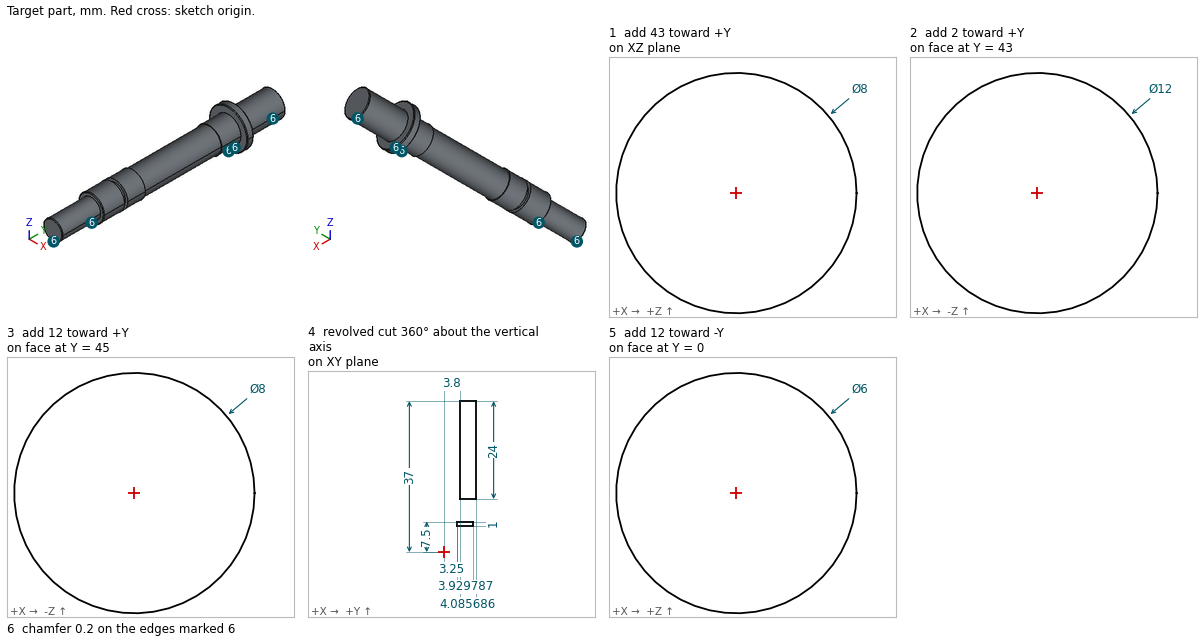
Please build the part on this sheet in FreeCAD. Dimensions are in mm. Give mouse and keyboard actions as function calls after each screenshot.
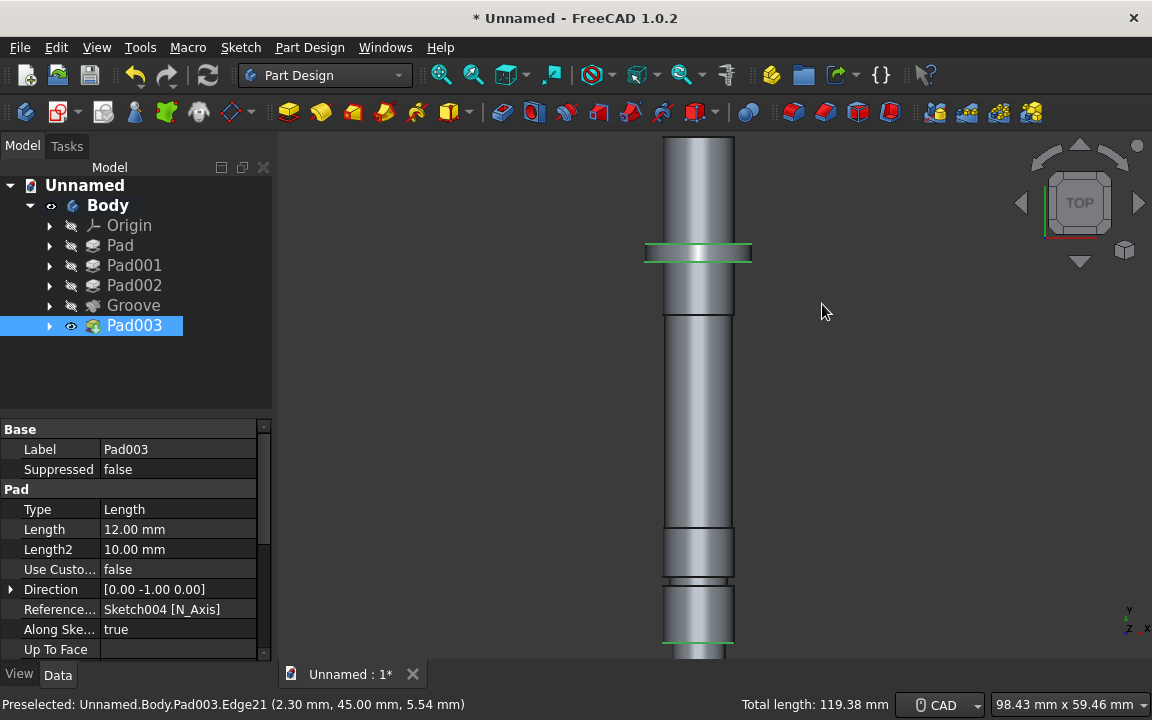
click(442, 76)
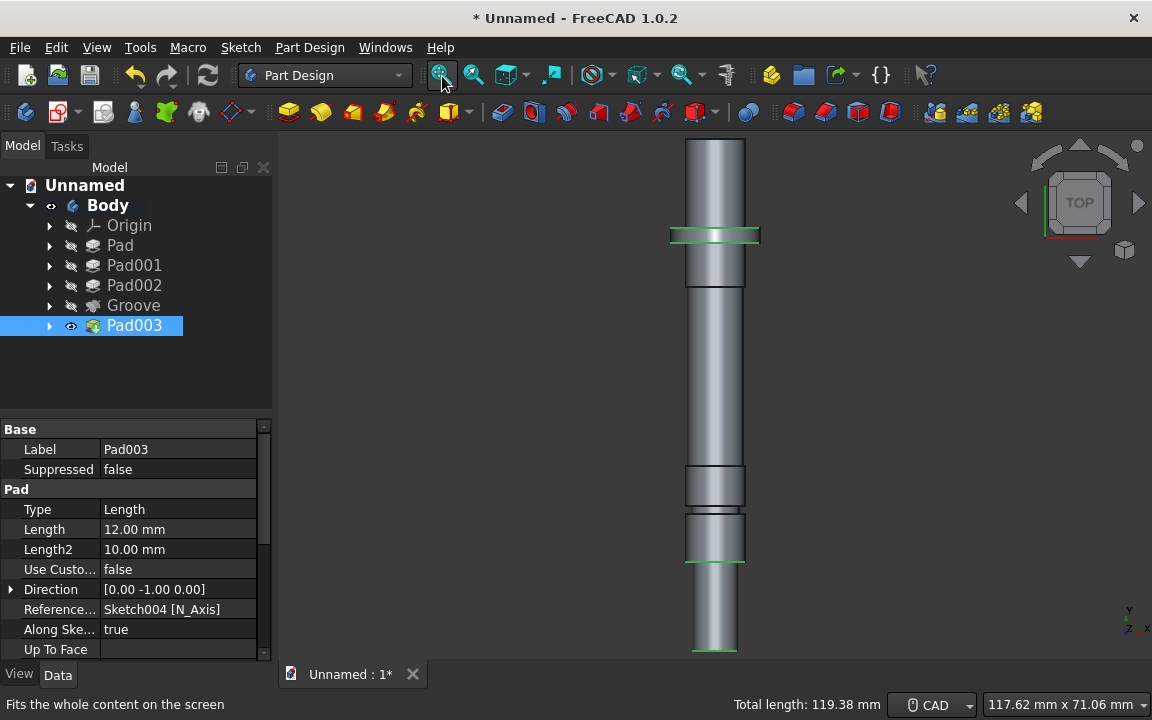
key(0)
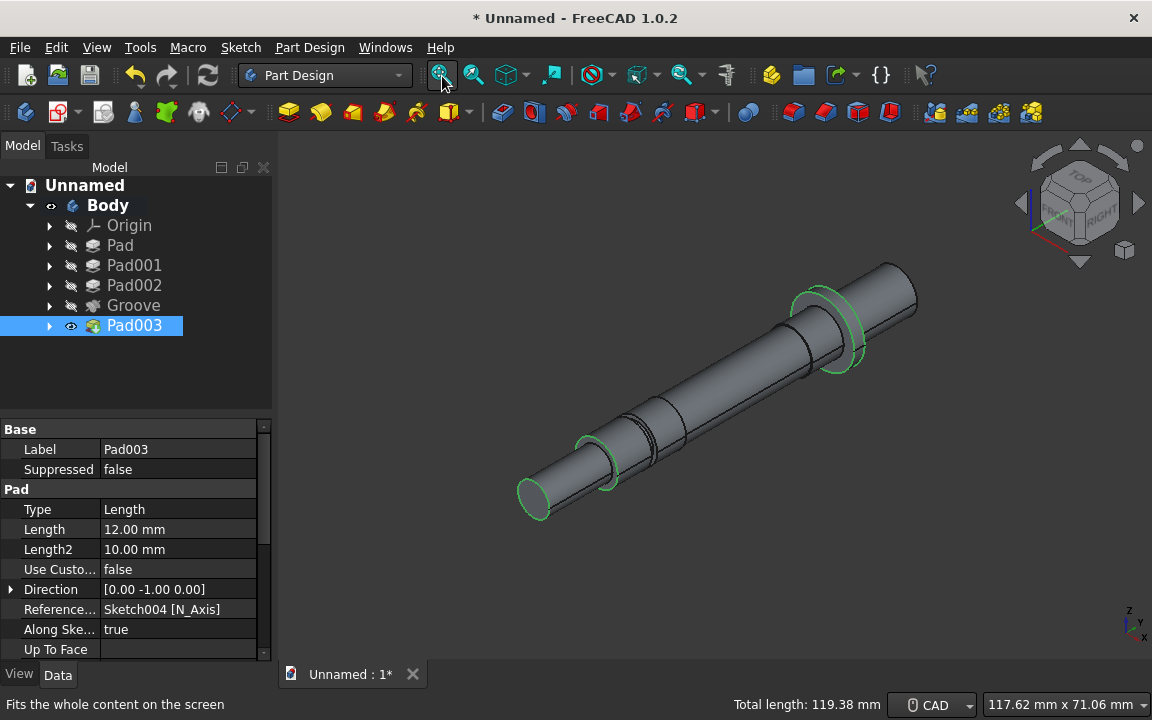
key(1)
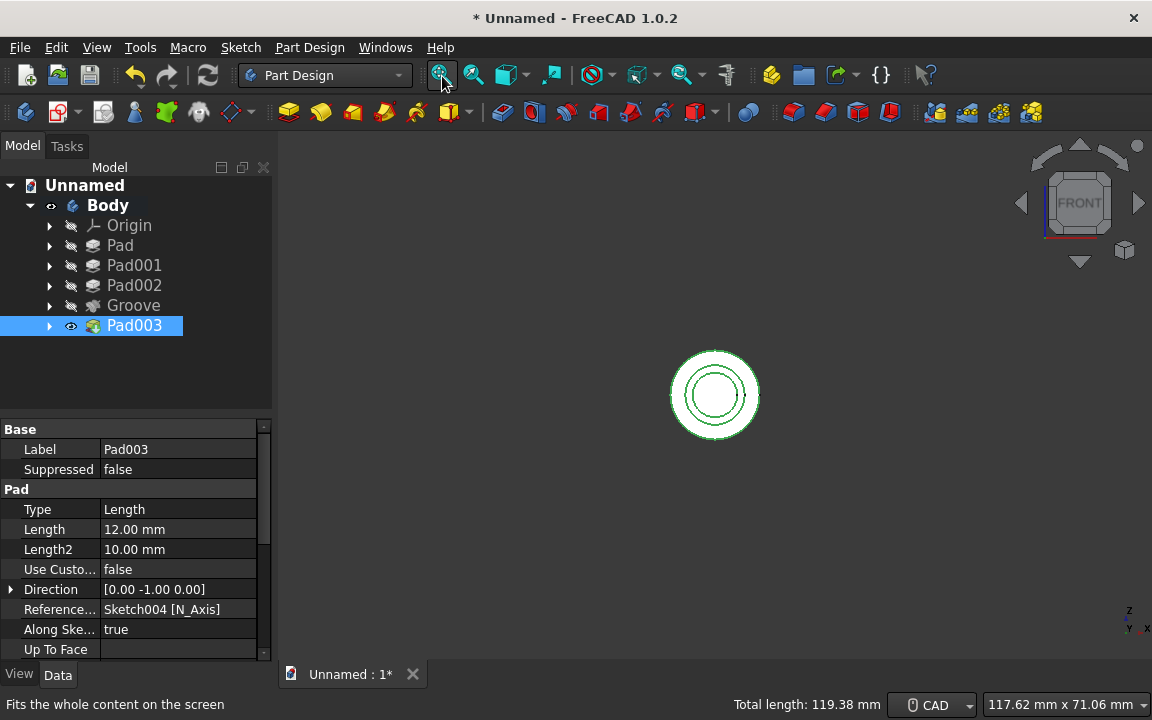
click(442, 76)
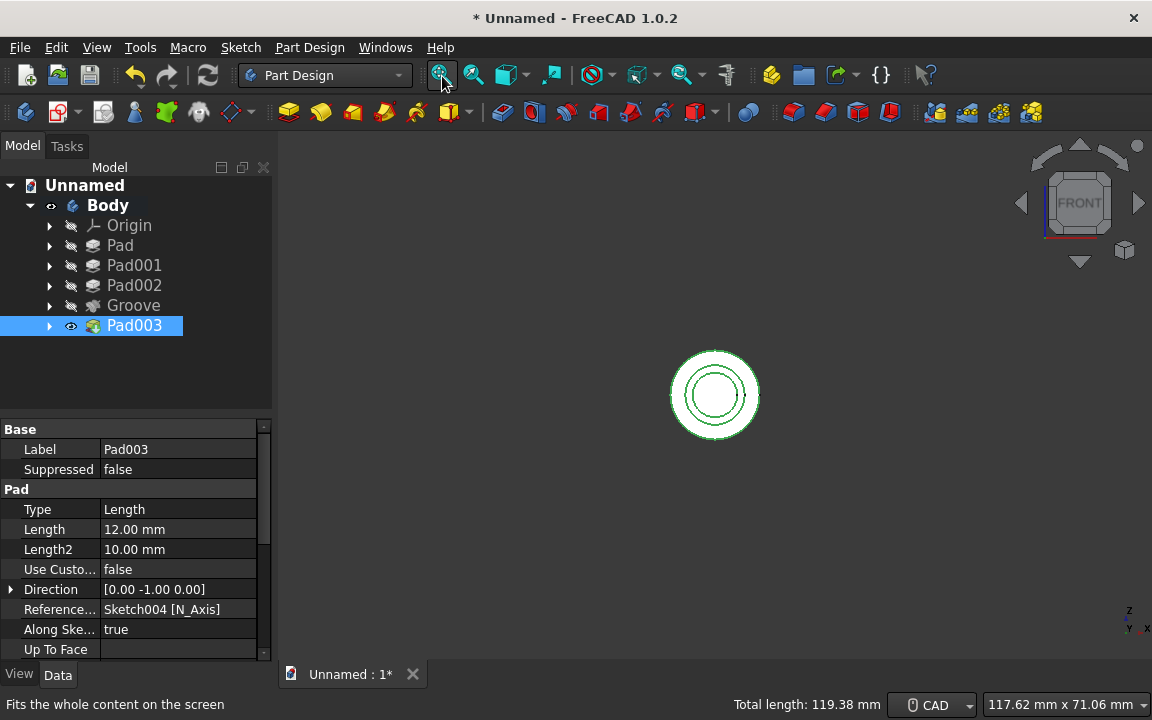
key(3)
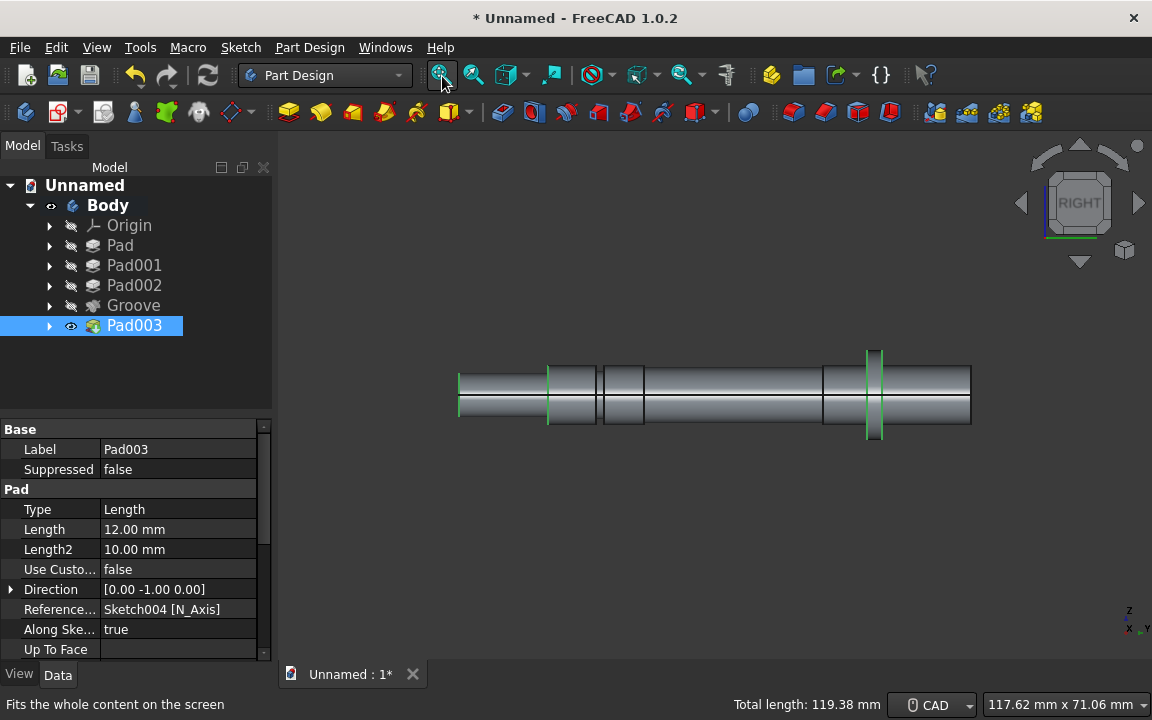
click(971, 411, ctrl)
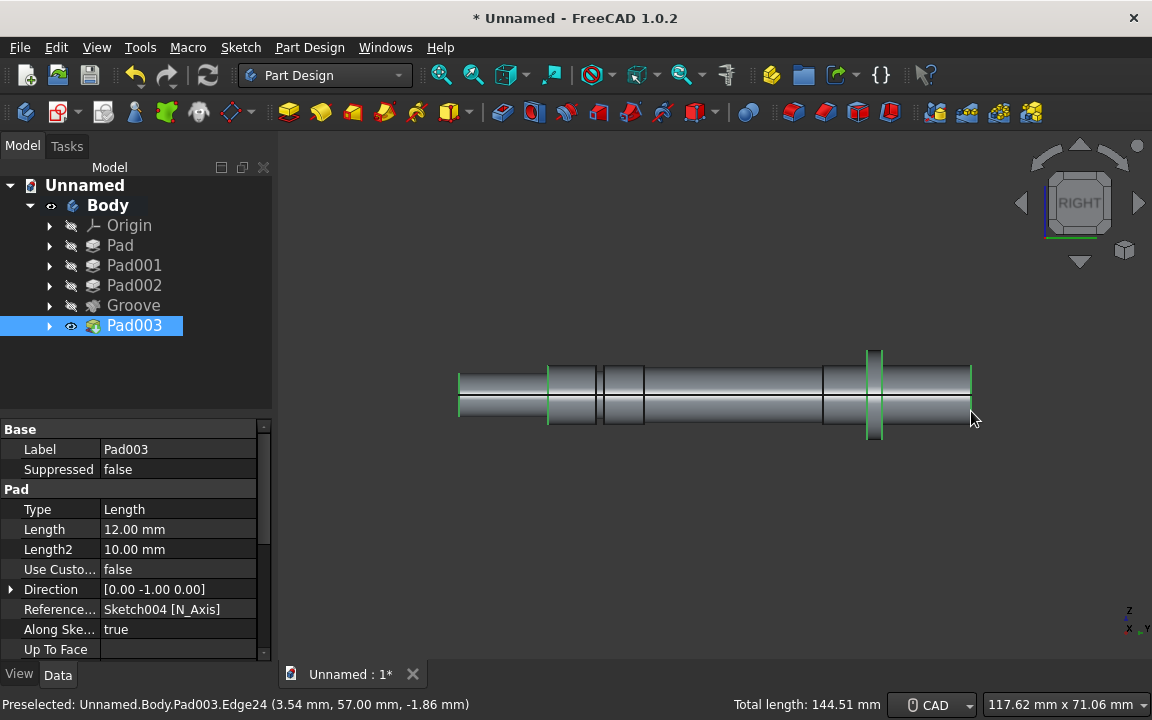
click(826, 112)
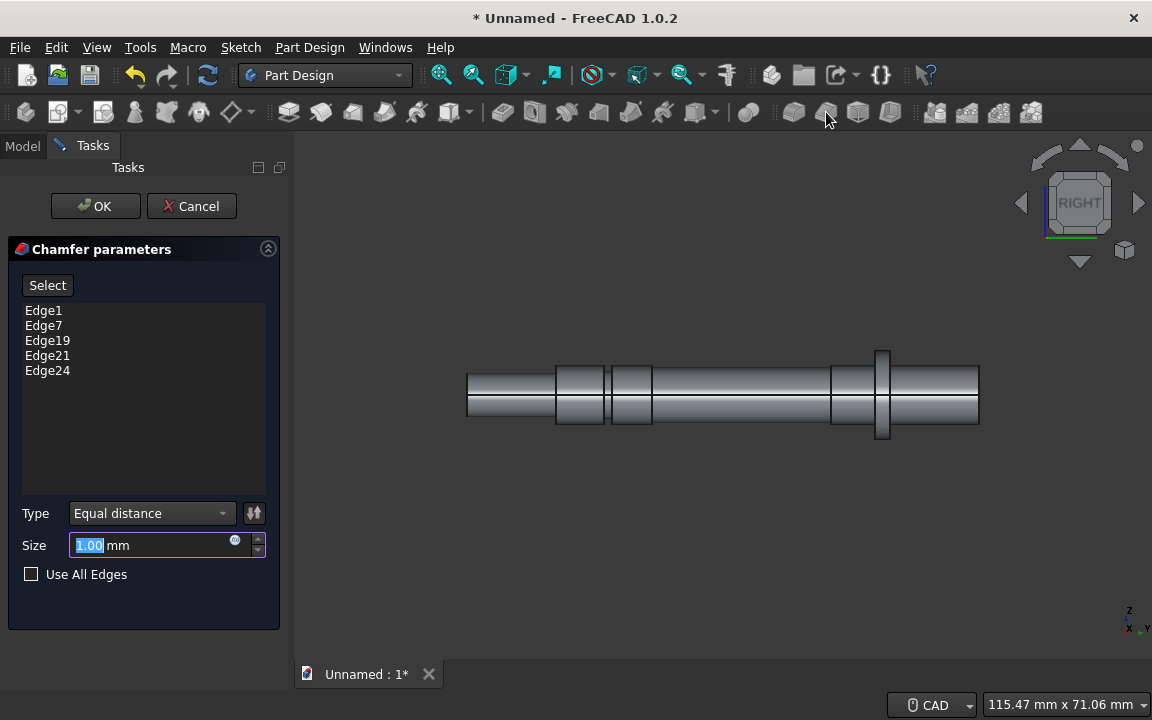
text(0.2)
key(Tab)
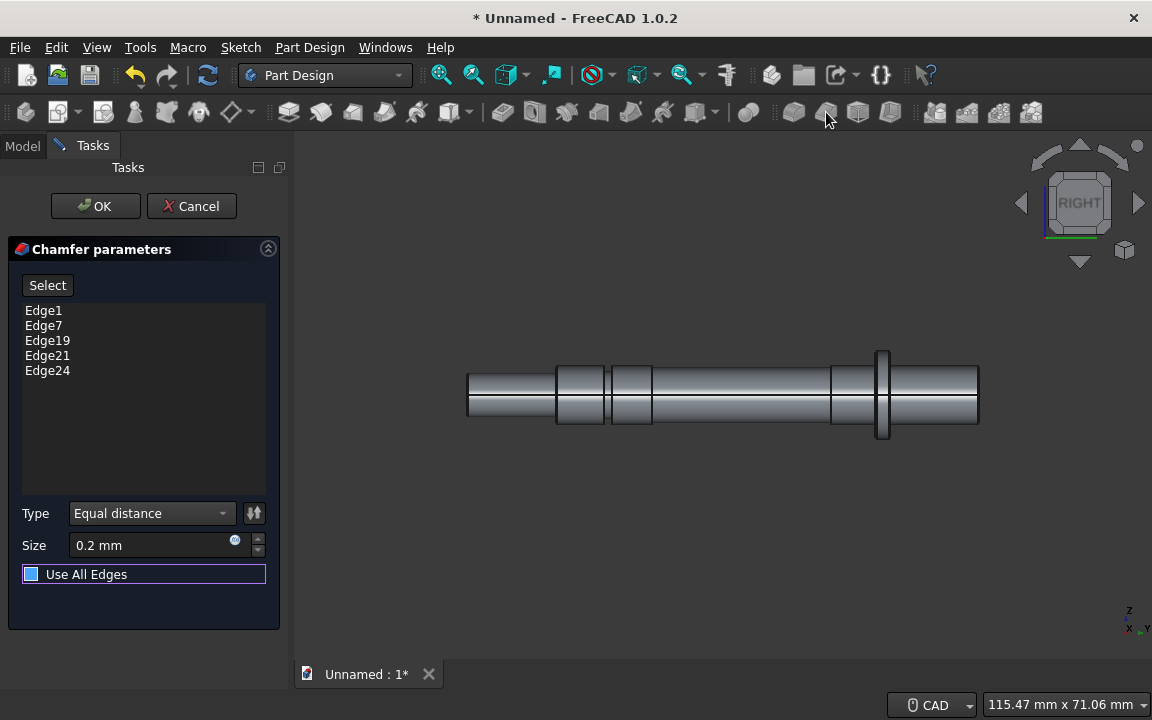
click(96, 206)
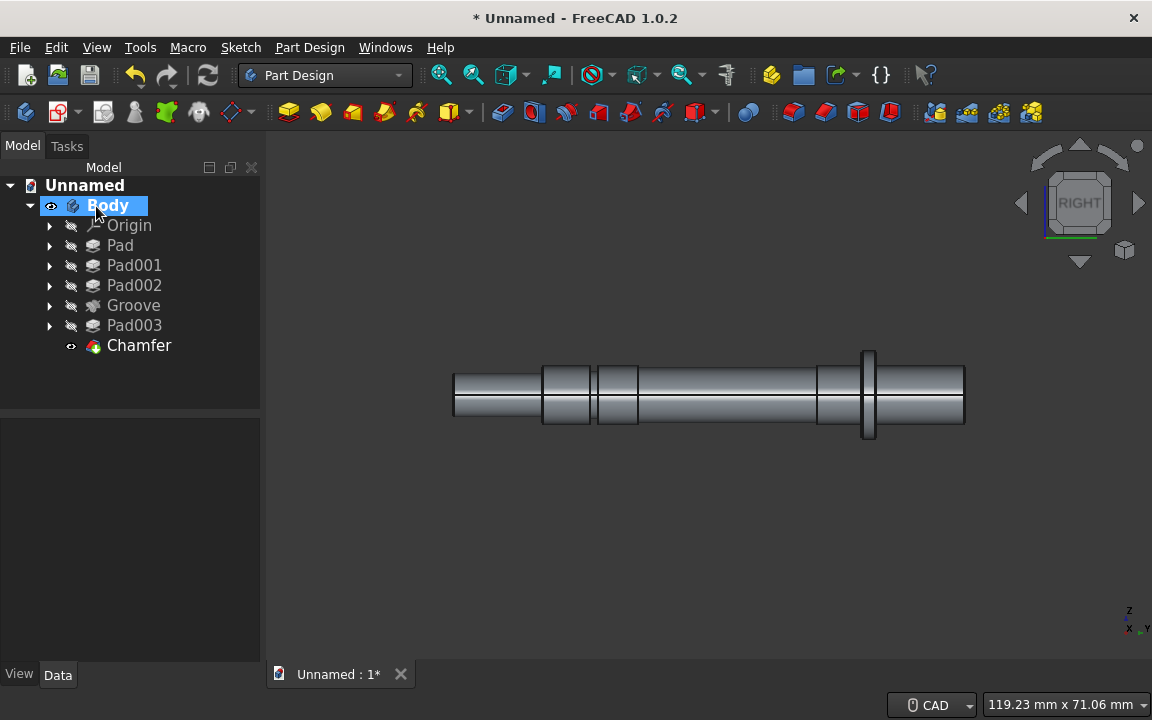
key(0)